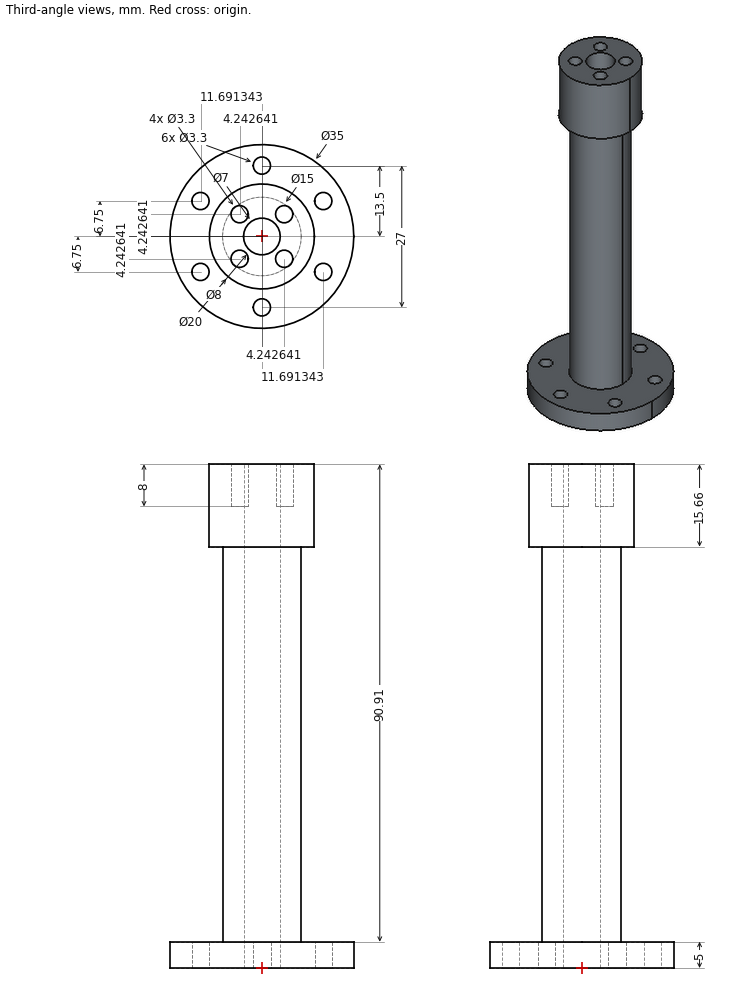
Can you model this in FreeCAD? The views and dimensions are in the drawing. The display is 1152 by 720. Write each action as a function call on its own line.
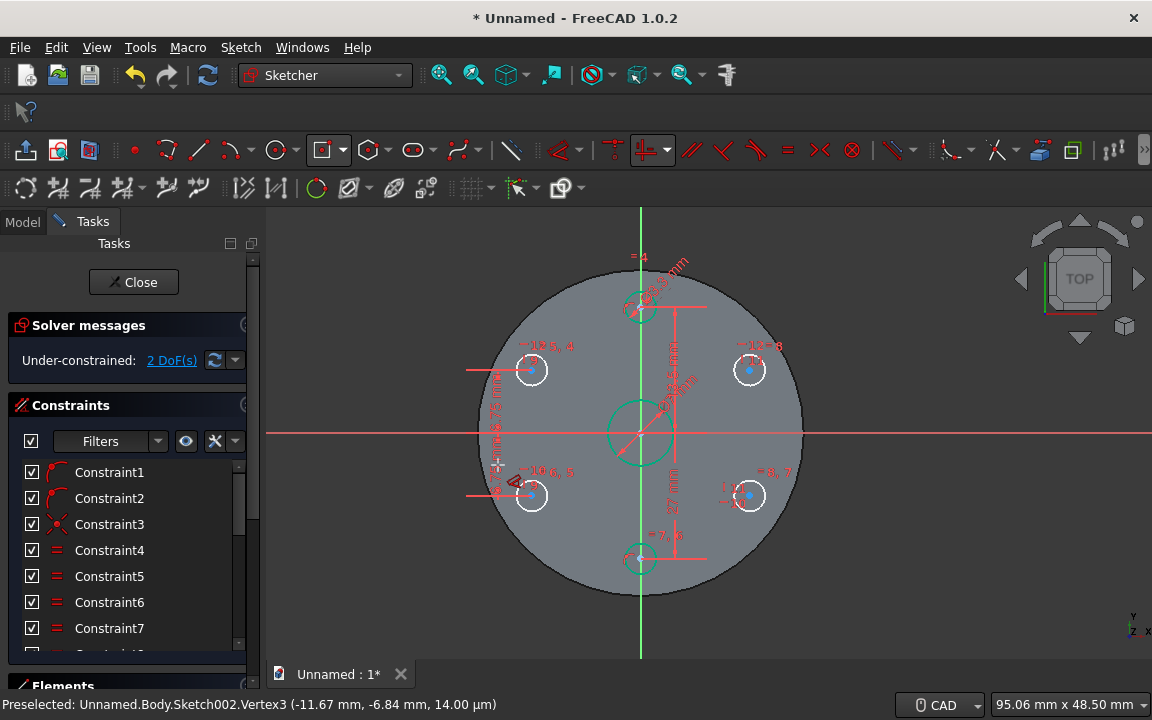
click(532, 370)
click(586, 336)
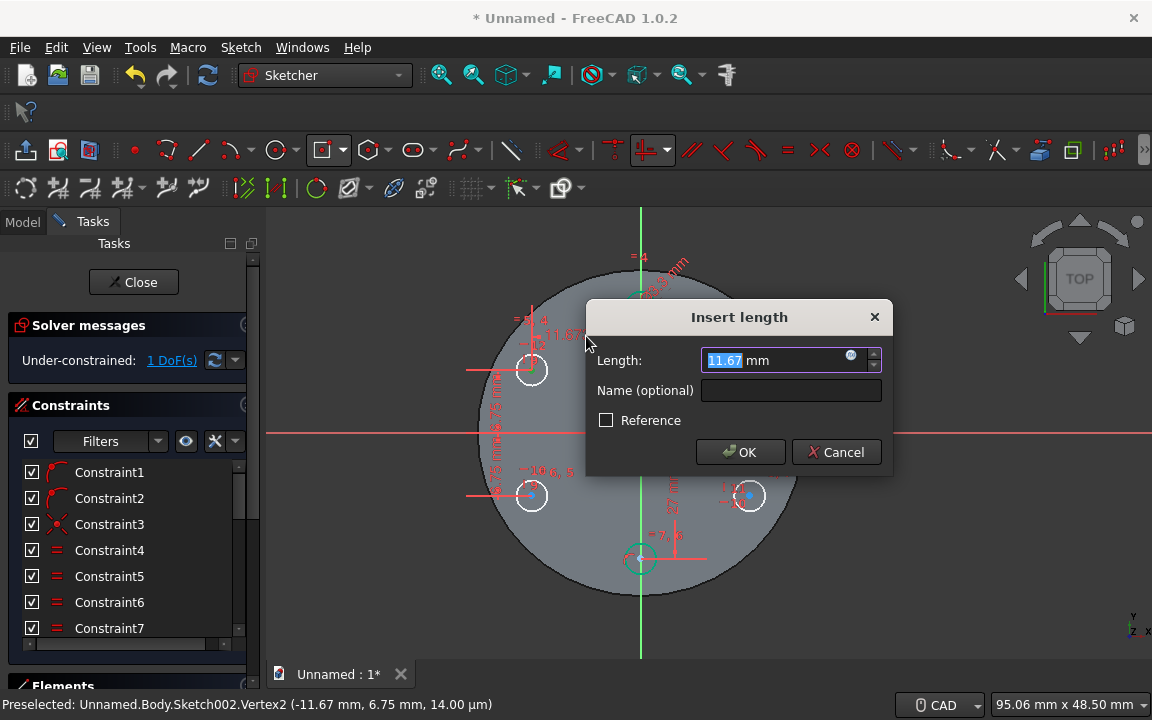
text(11.691343)
key(Return)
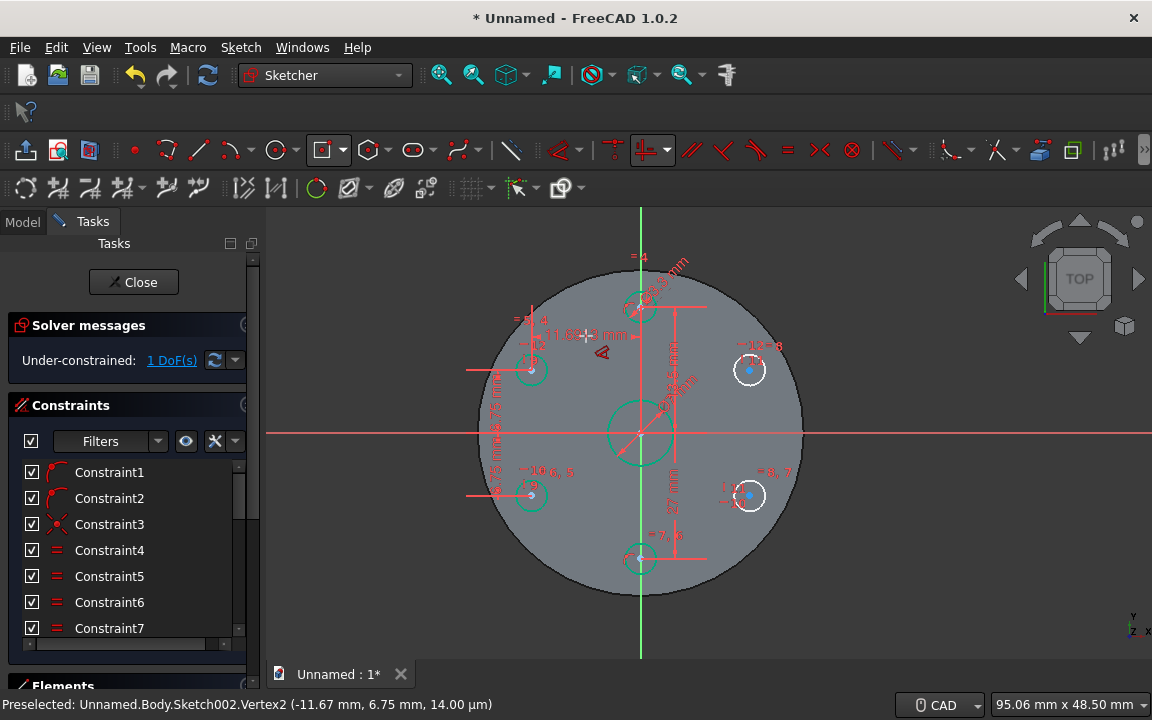
click(750, 496)
click(695, 530)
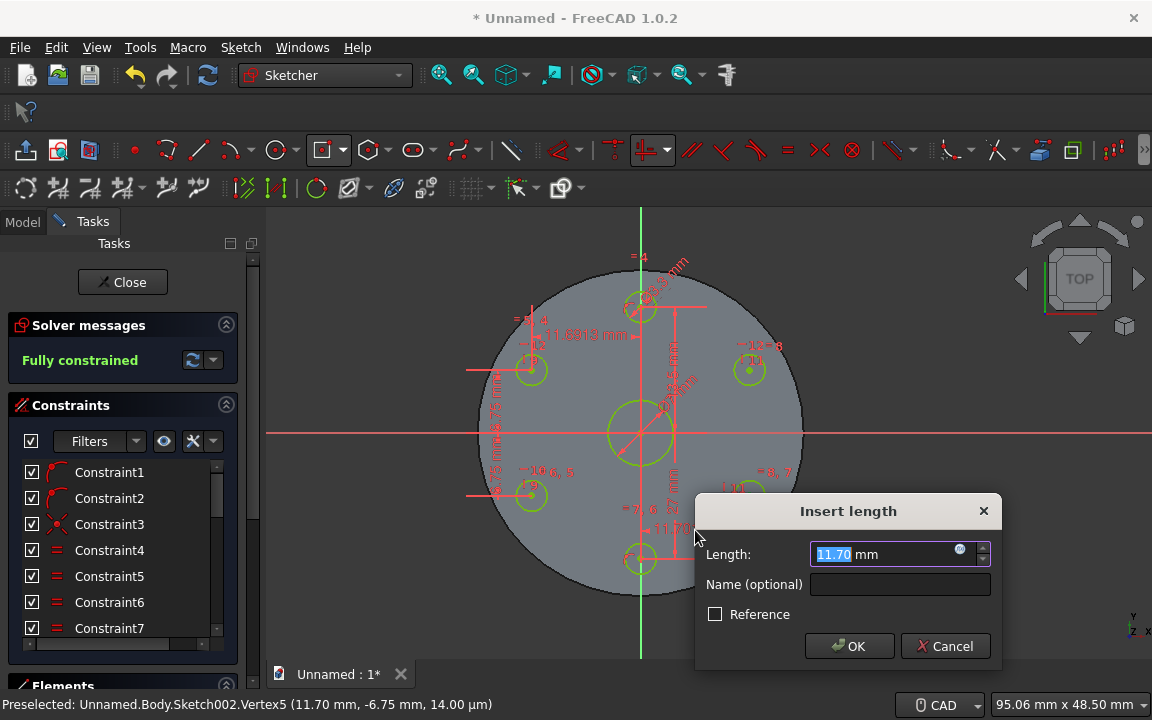
text(11.691343)
key(Return)
key(Escape)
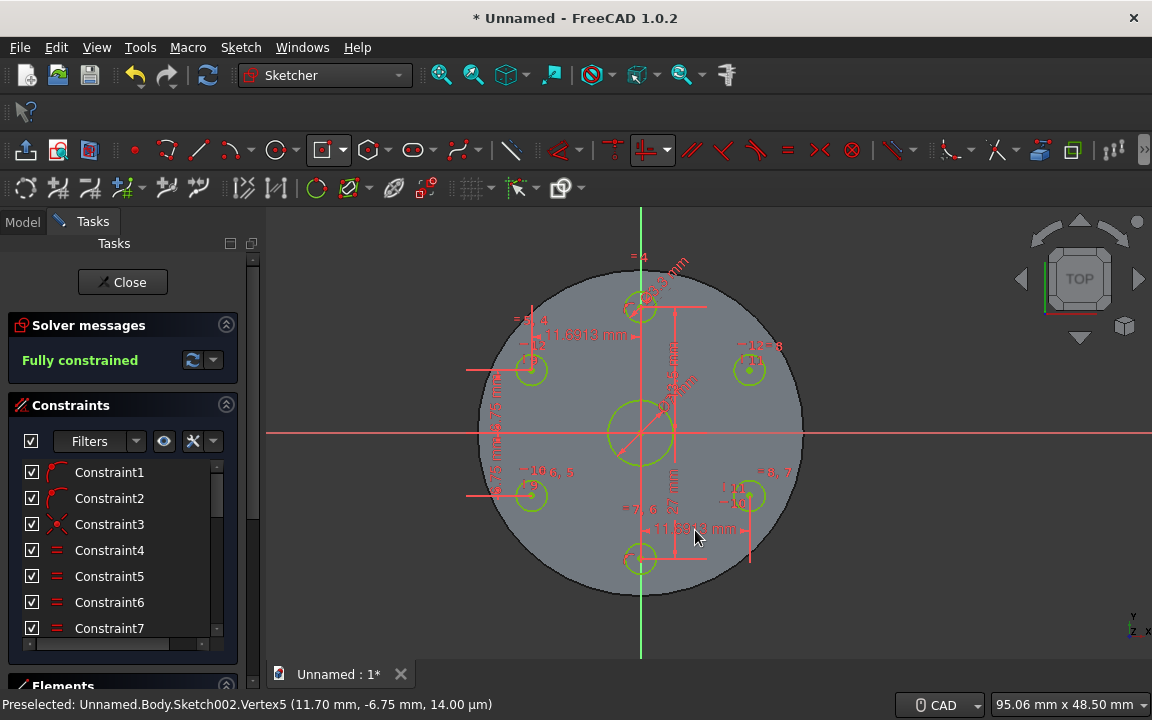
click(123, 282)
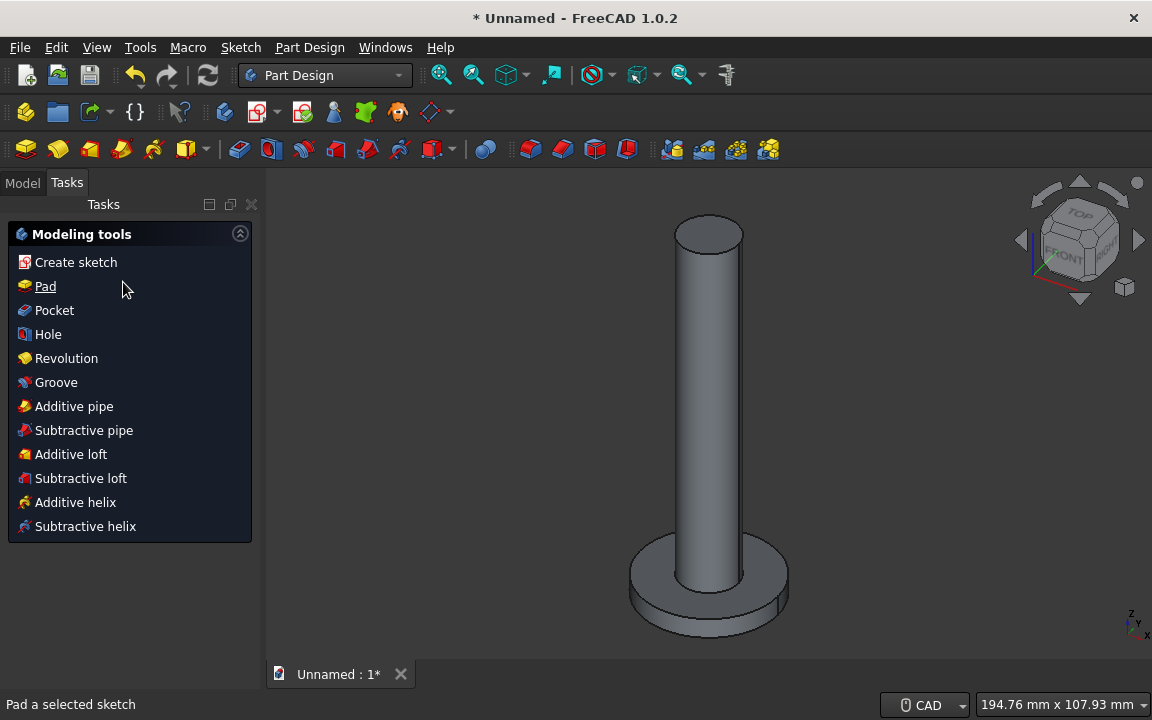
click(240, 150)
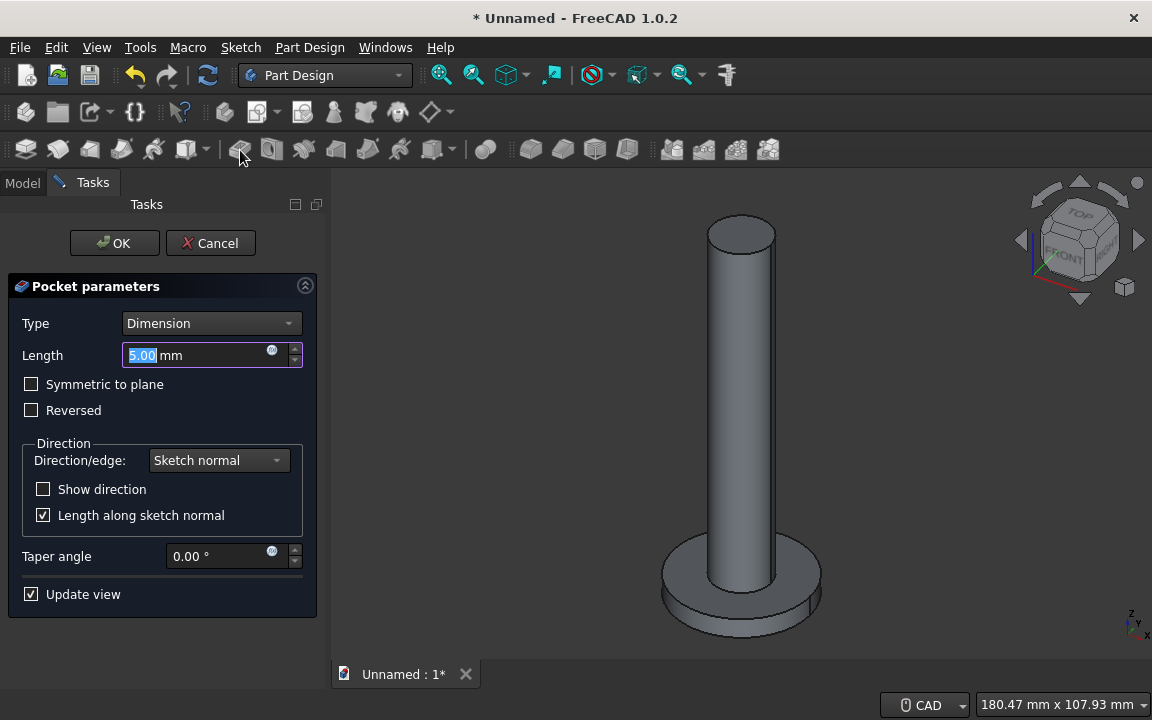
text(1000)
key(Tab)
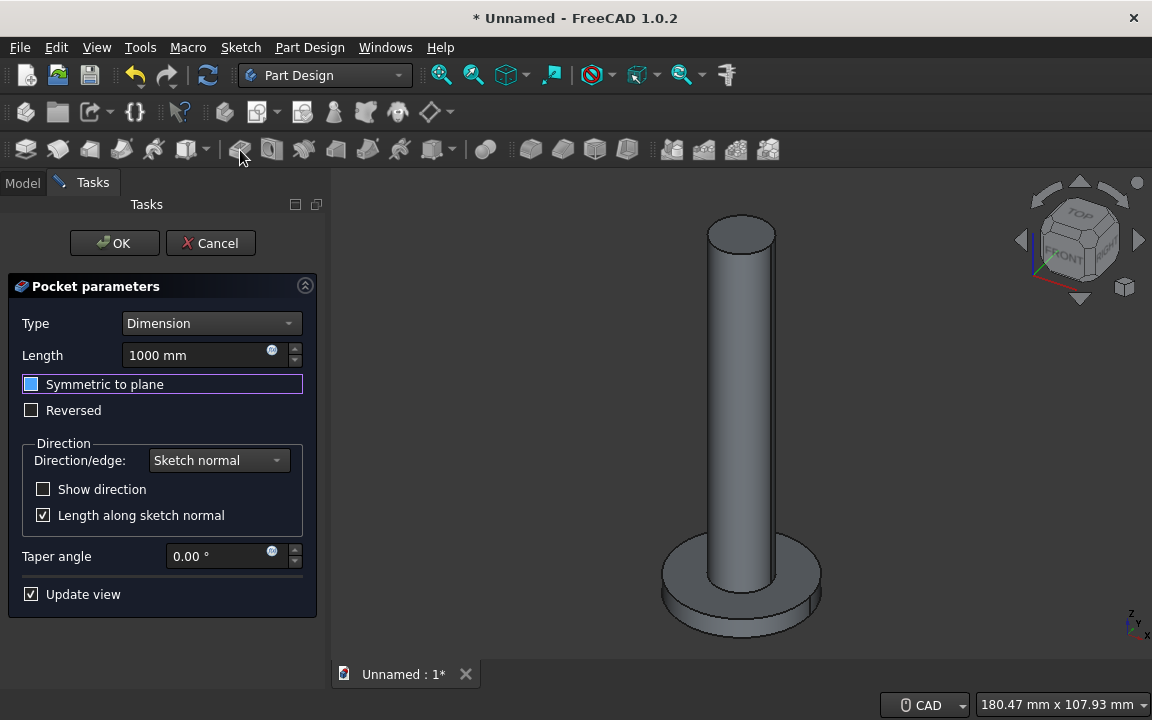
click(30, 410)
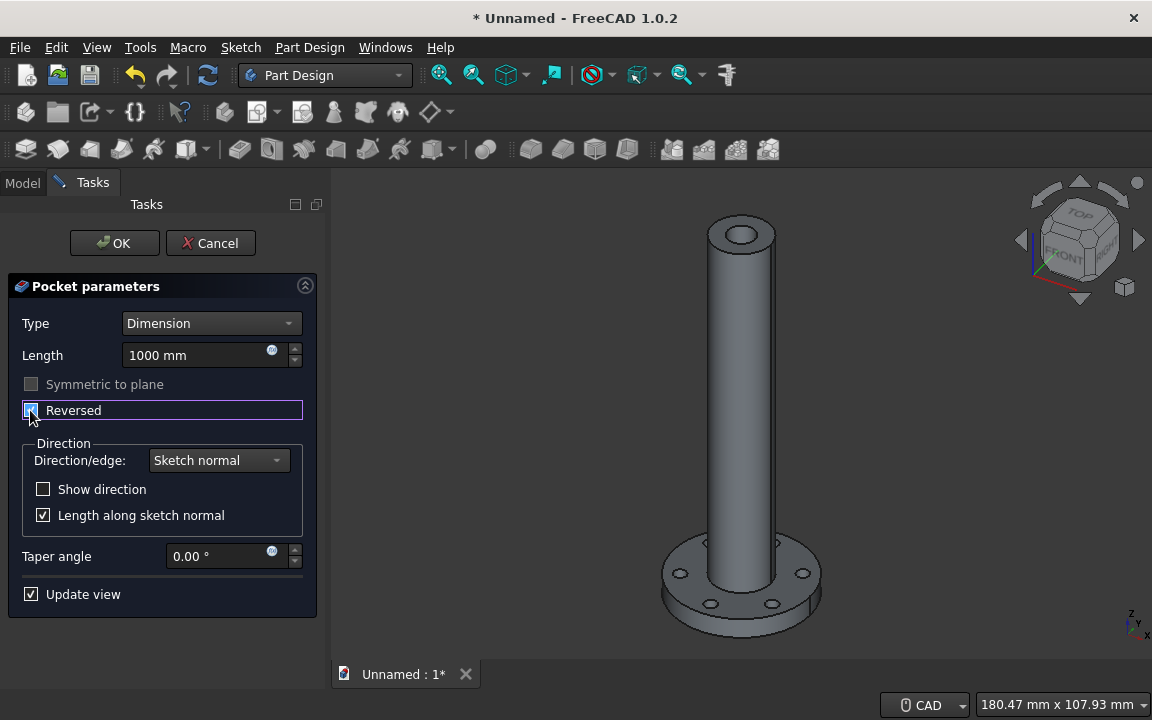
click(115, 243)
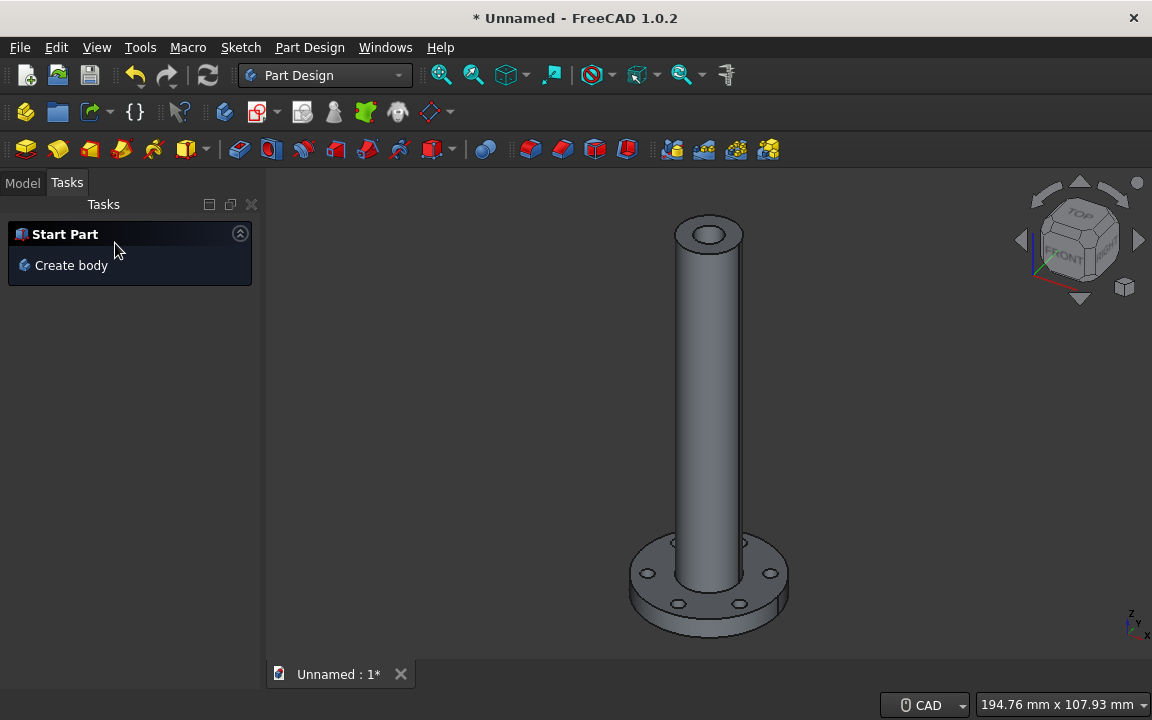
scroll(682, 238, up, 4)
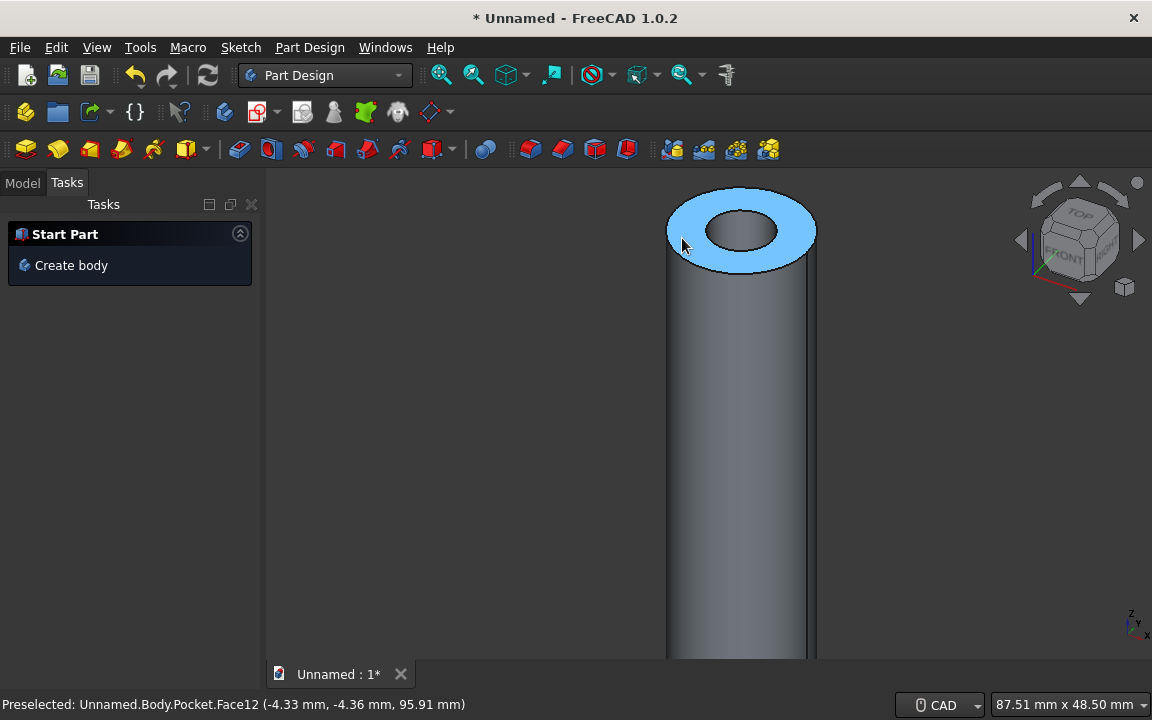
click(682, 239)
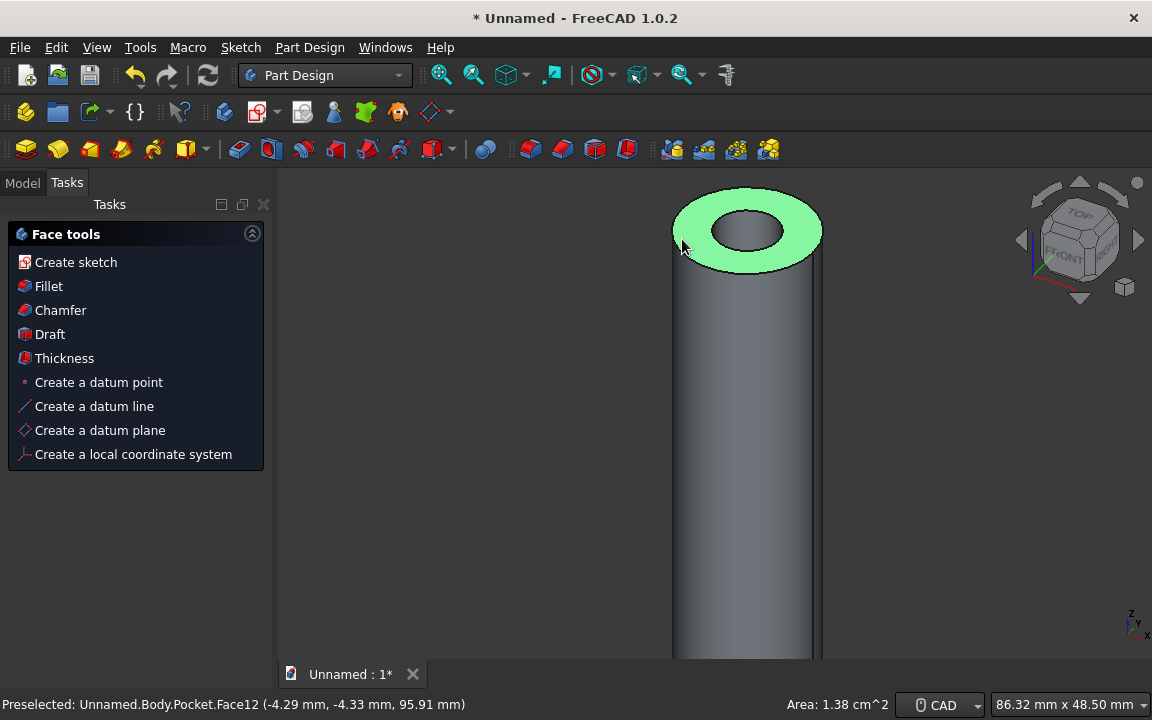
click(258, 112)